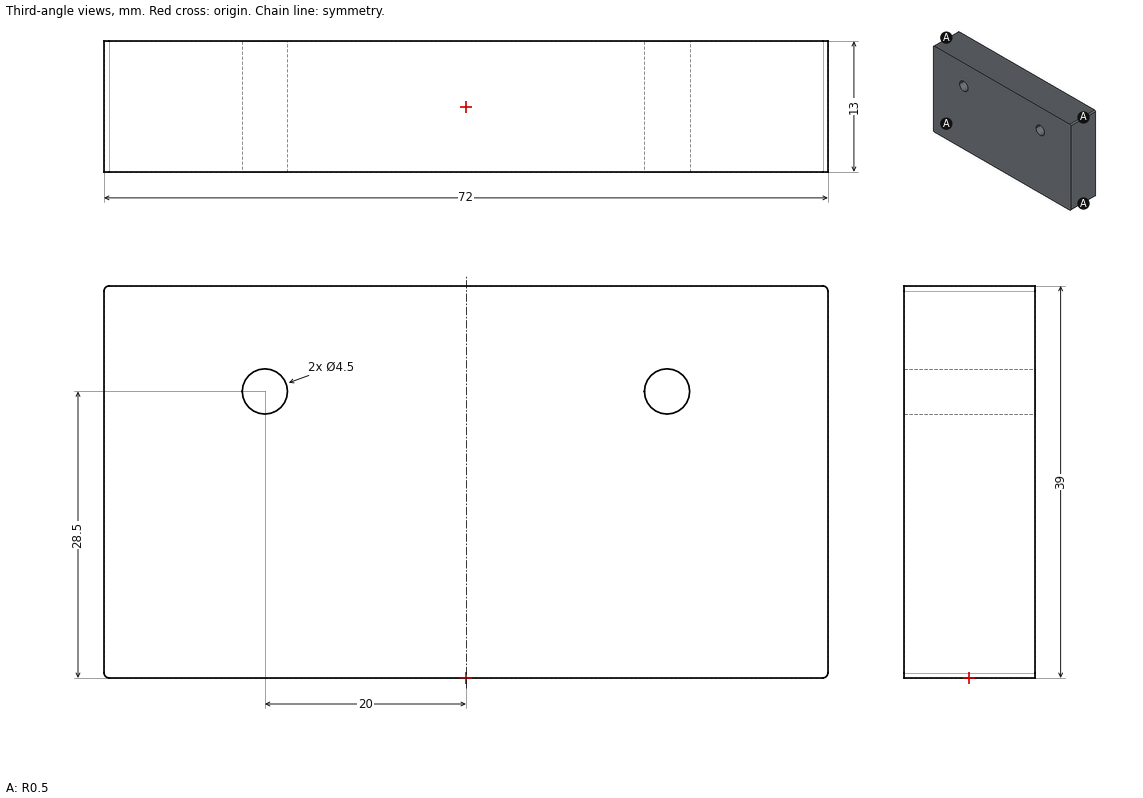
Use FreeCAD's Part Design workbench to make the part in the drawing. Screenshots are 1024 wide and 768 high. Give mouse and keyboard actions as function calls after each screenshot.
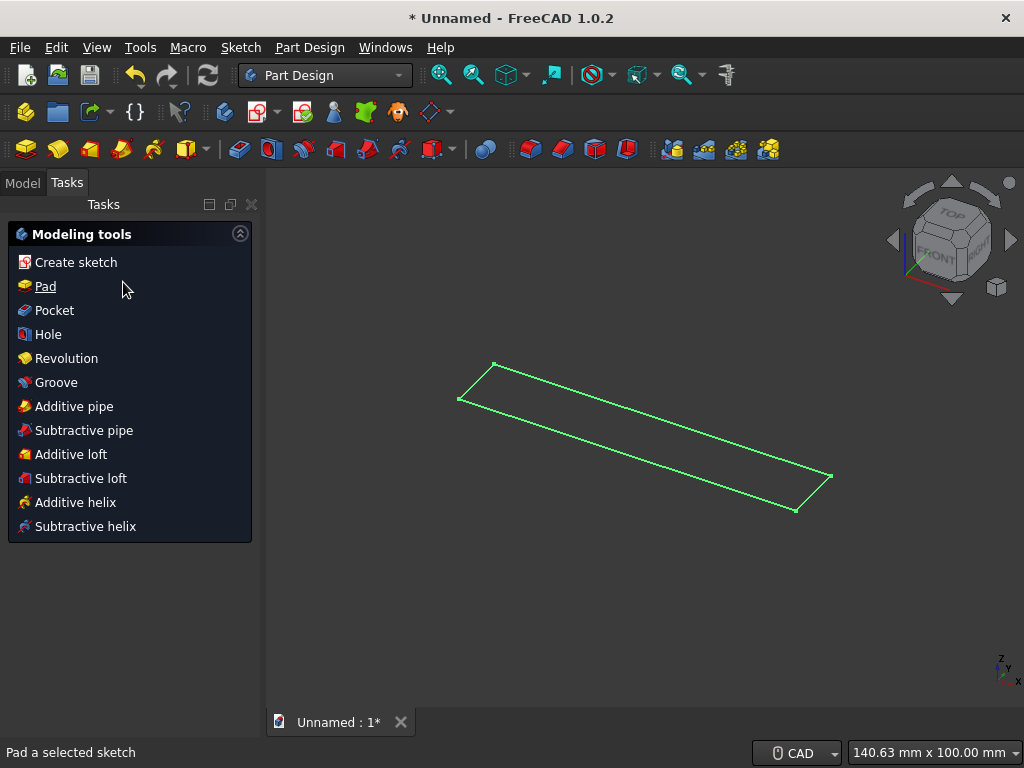
click(26, 150)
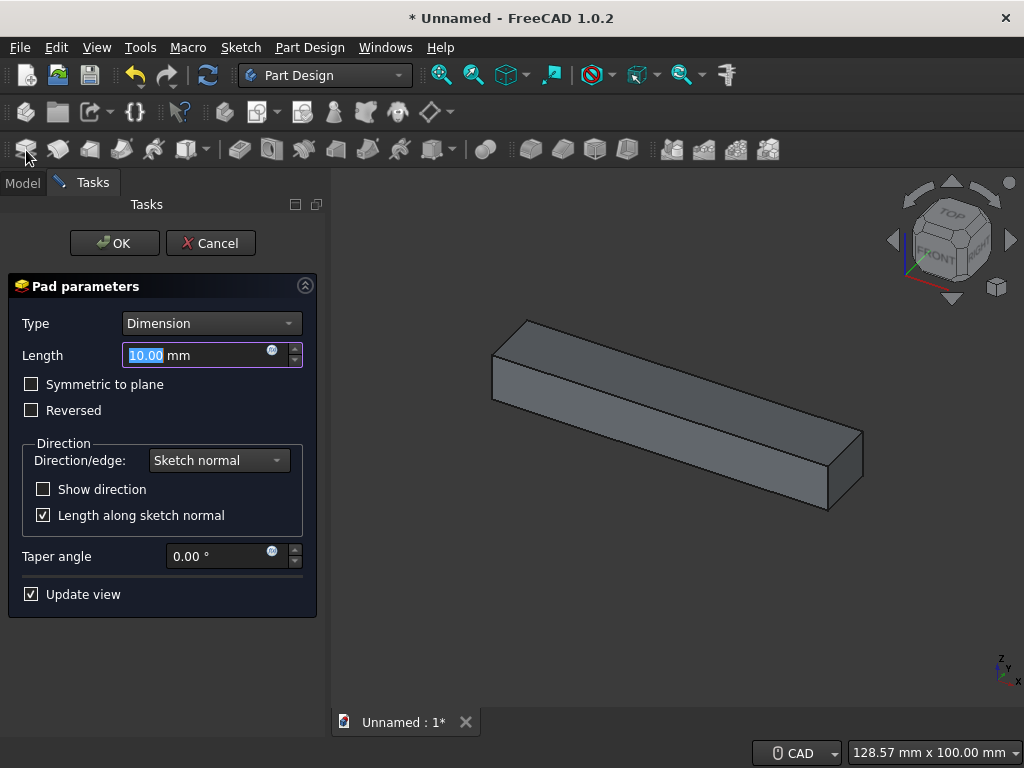
text(39)
key(Tab)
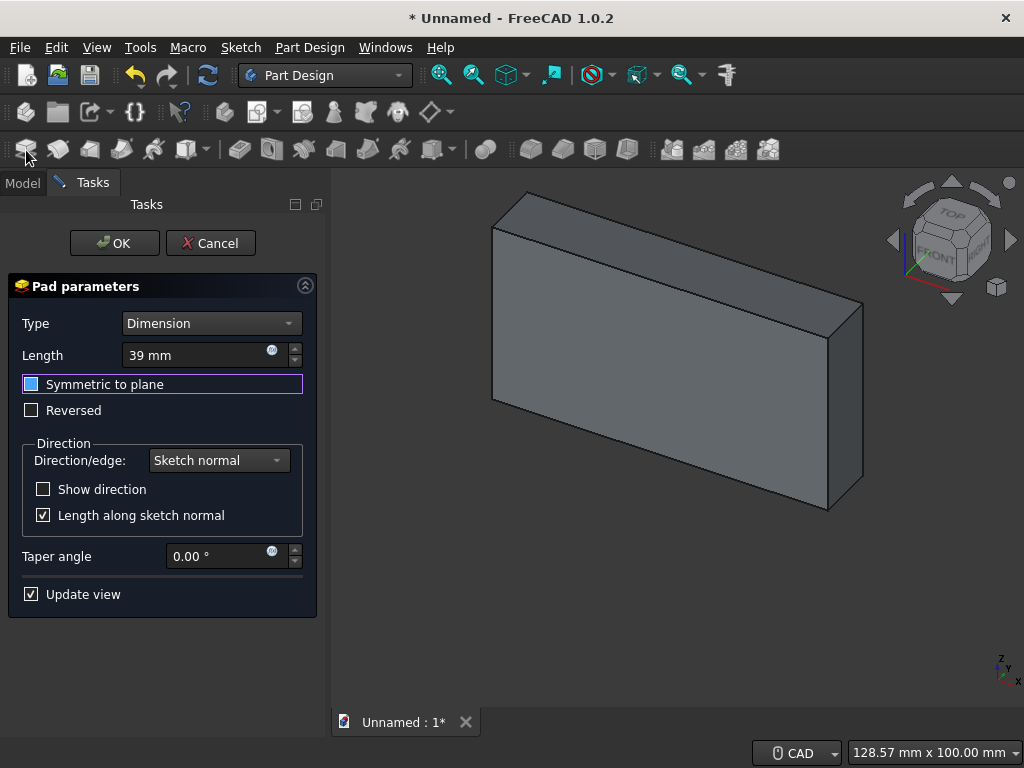
click(115, 243)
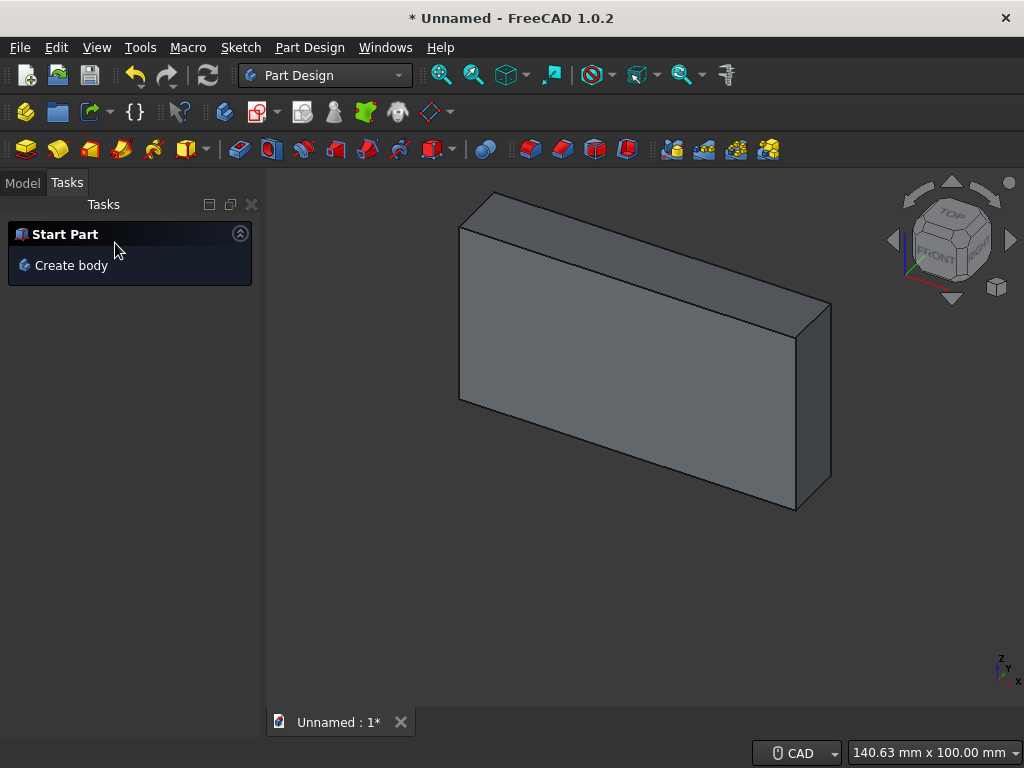
click(813, 320)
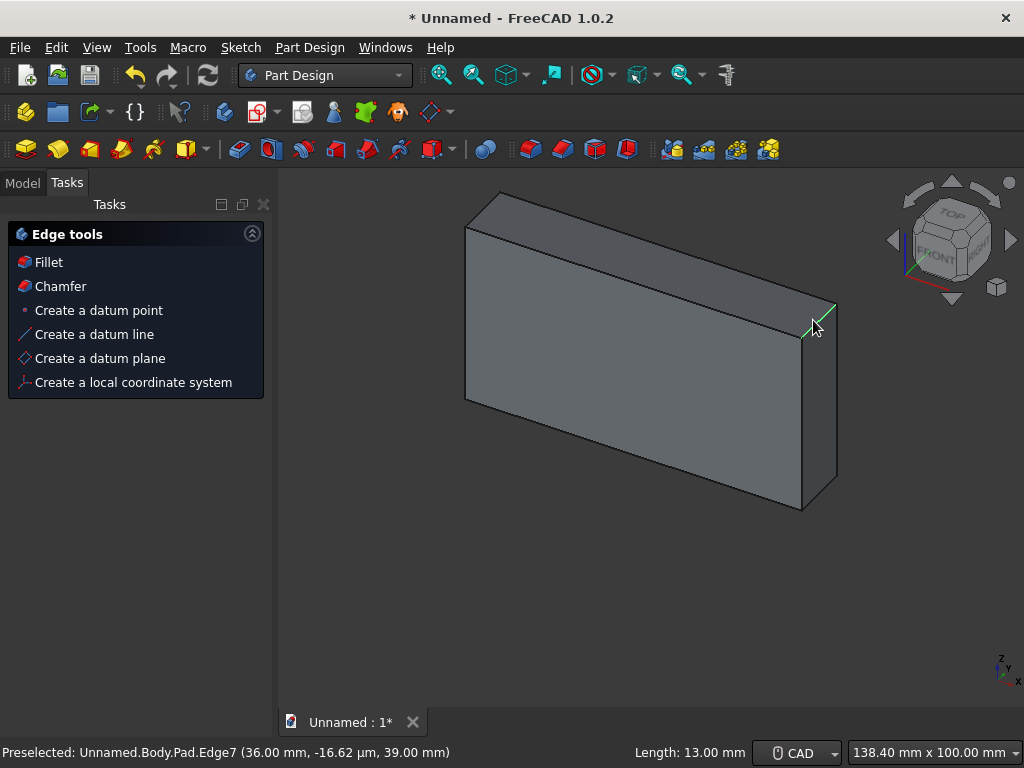
key(0)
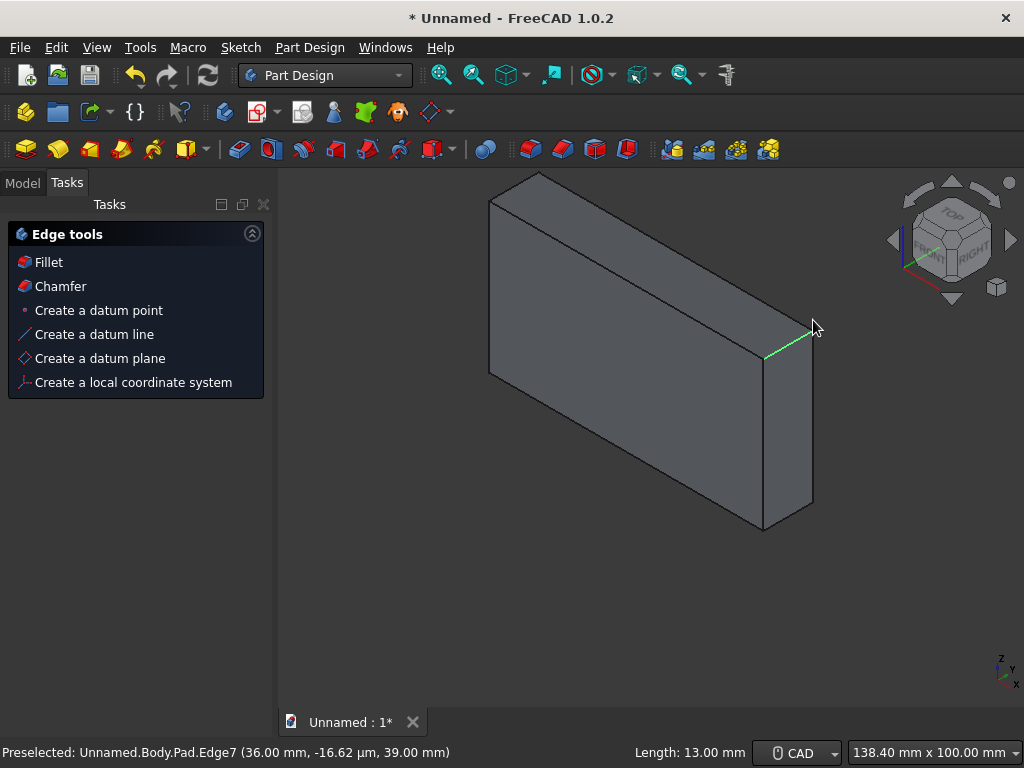
key(2)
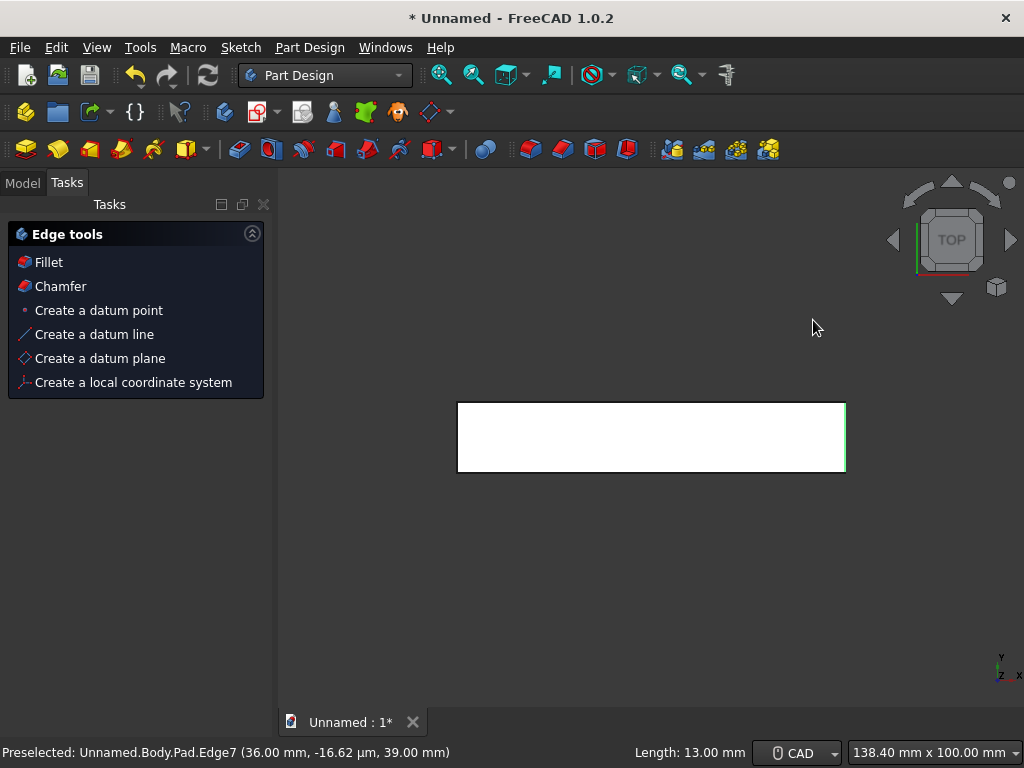
click(457, 436, ctrl)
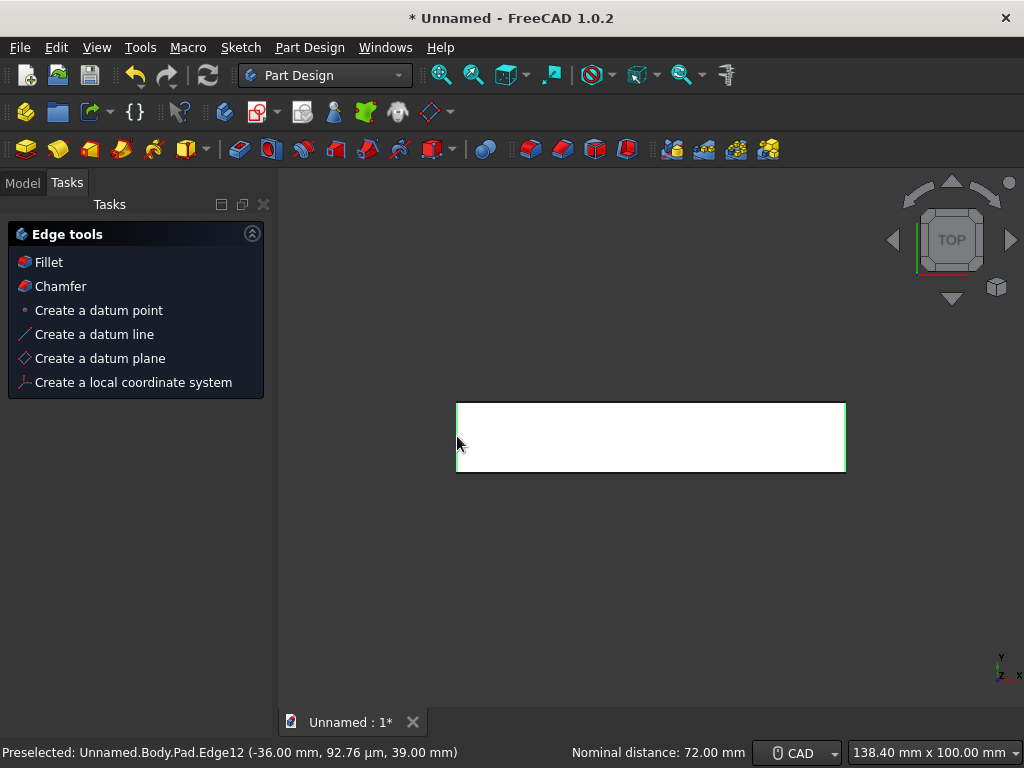
key(1)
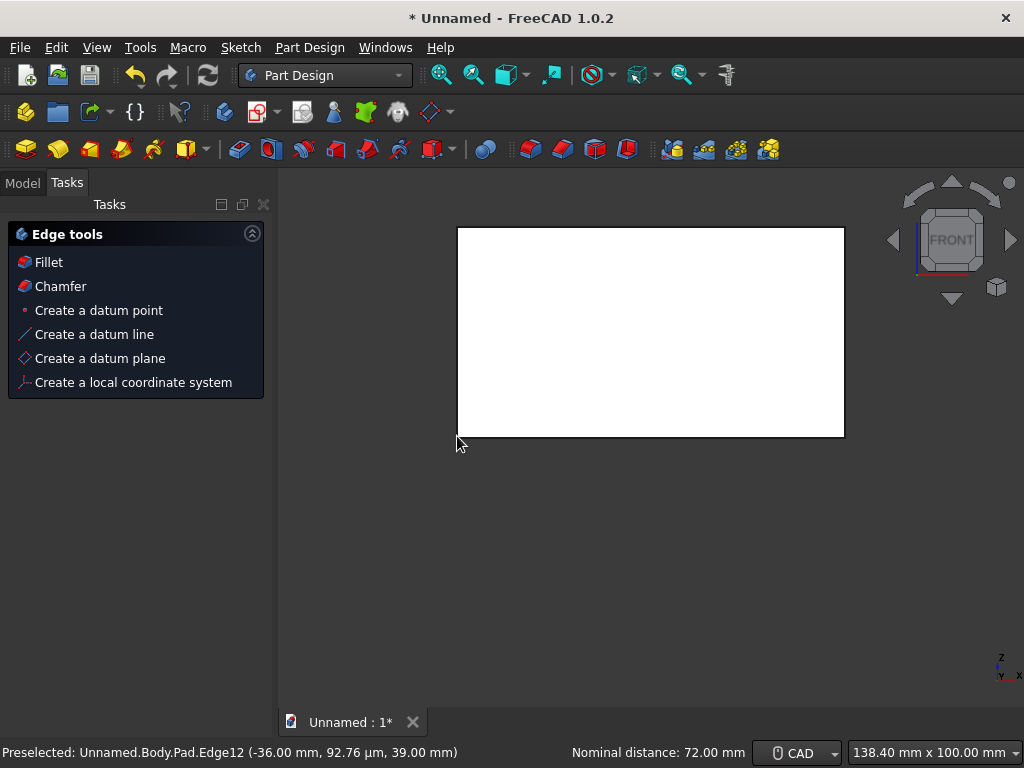
key(3)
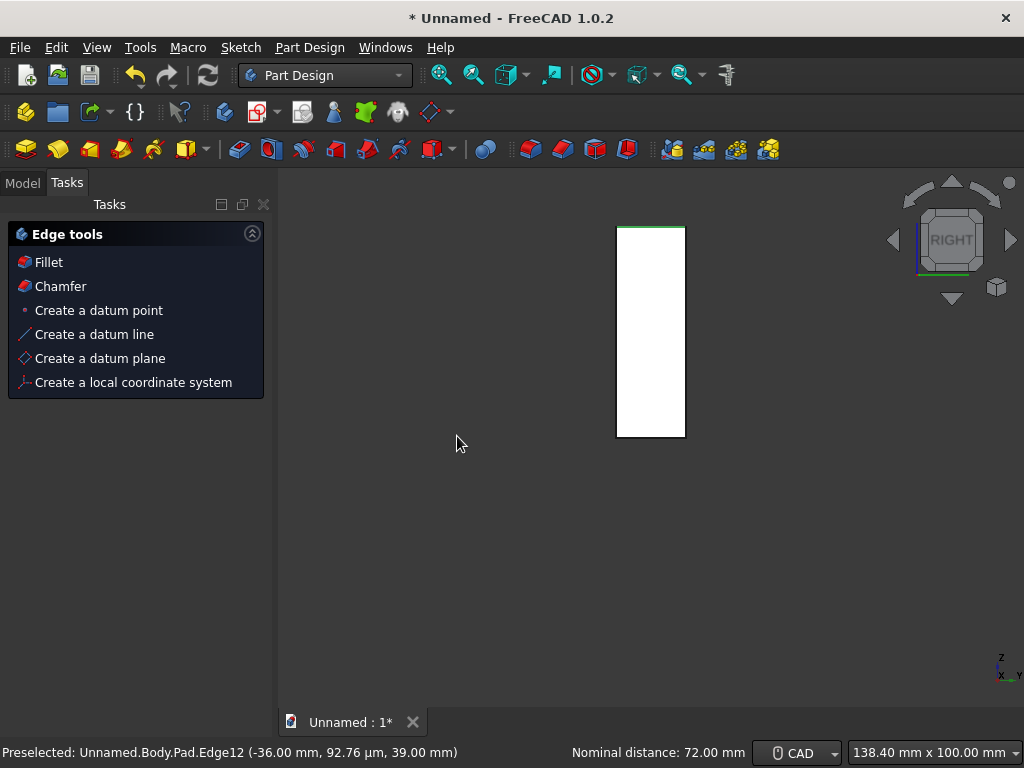
click(442, 76)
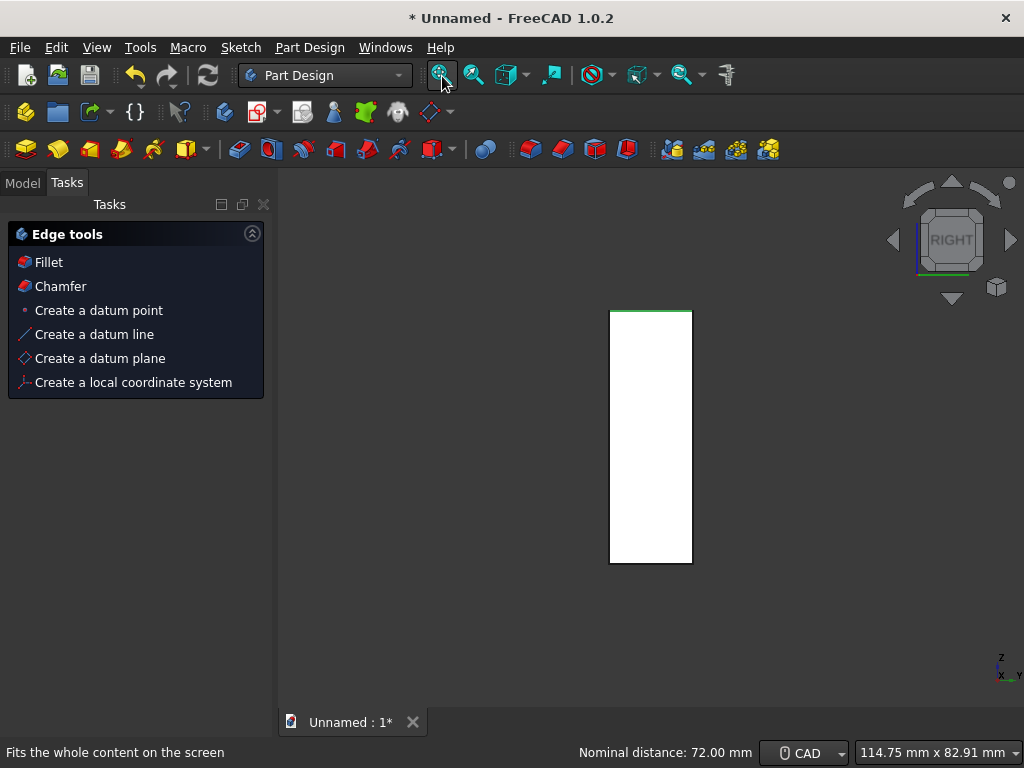
click(651, 563, ctrl)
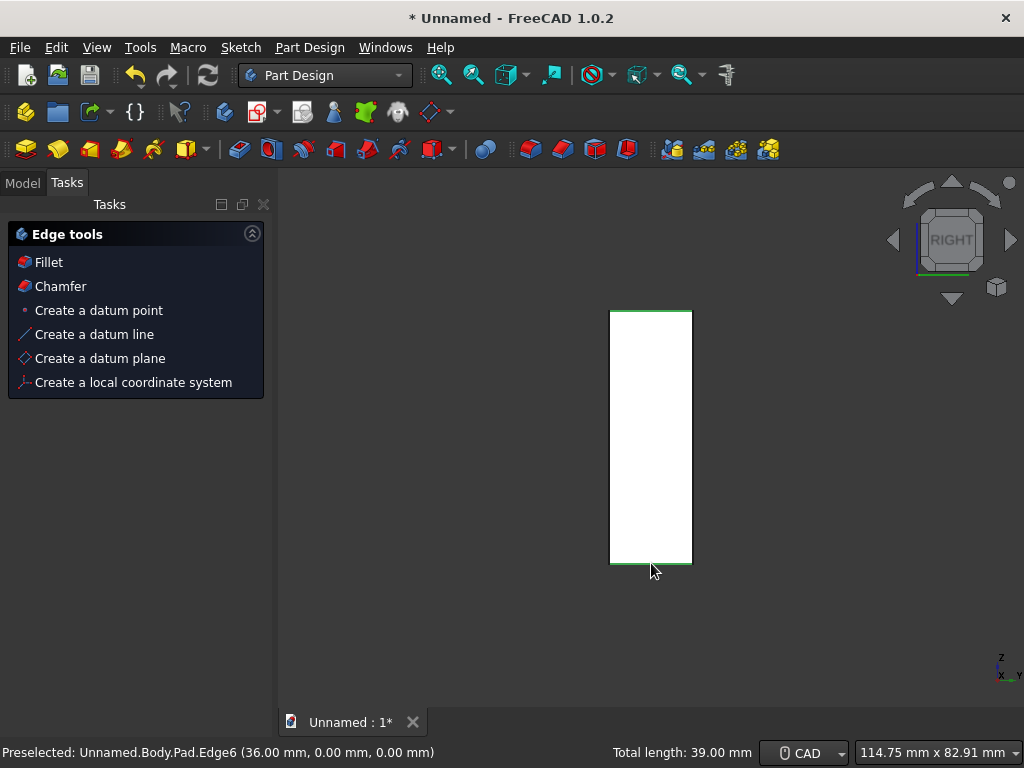
key(5)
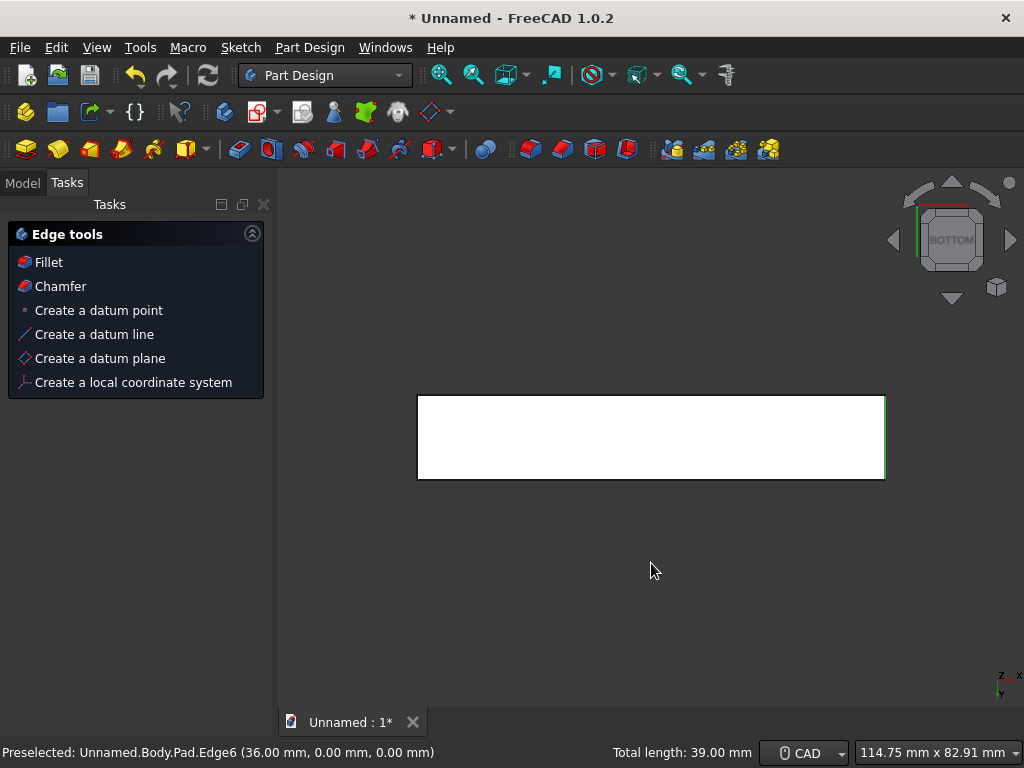
click(417, 436, ctrl)